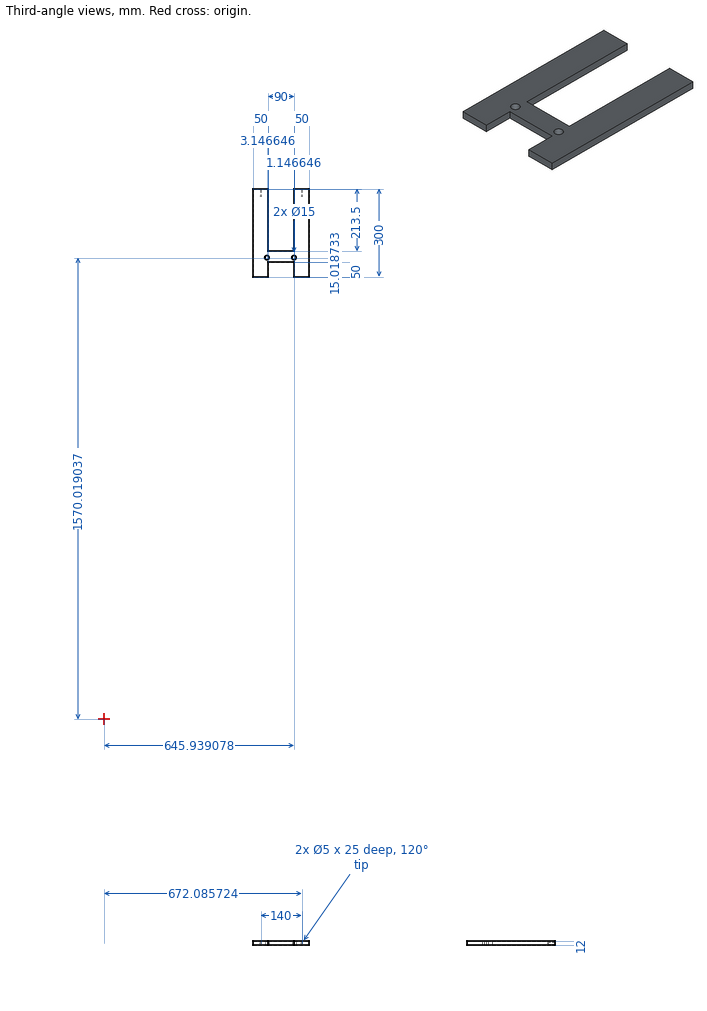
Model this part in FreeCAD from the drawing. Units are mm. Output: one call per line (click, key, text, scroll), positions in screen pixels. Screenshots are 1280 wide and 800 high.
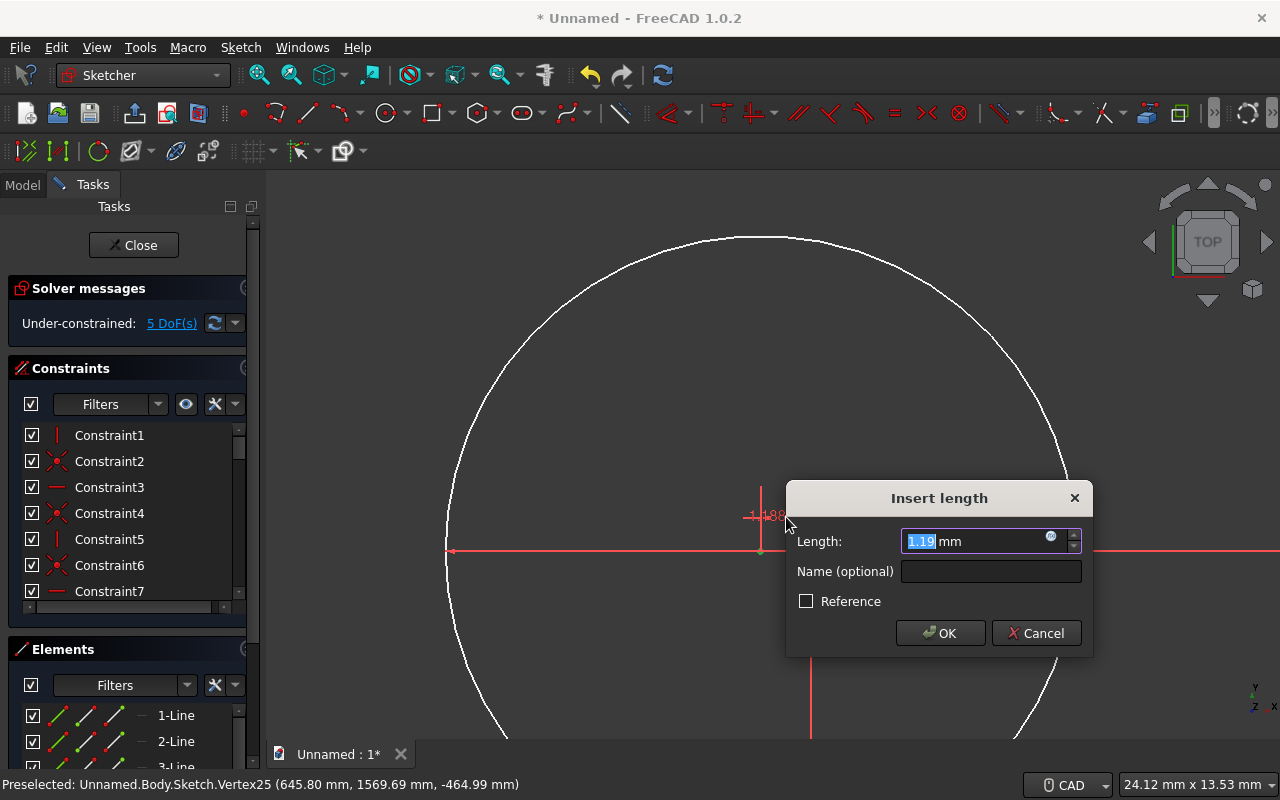
text(1.146646)
key(Return)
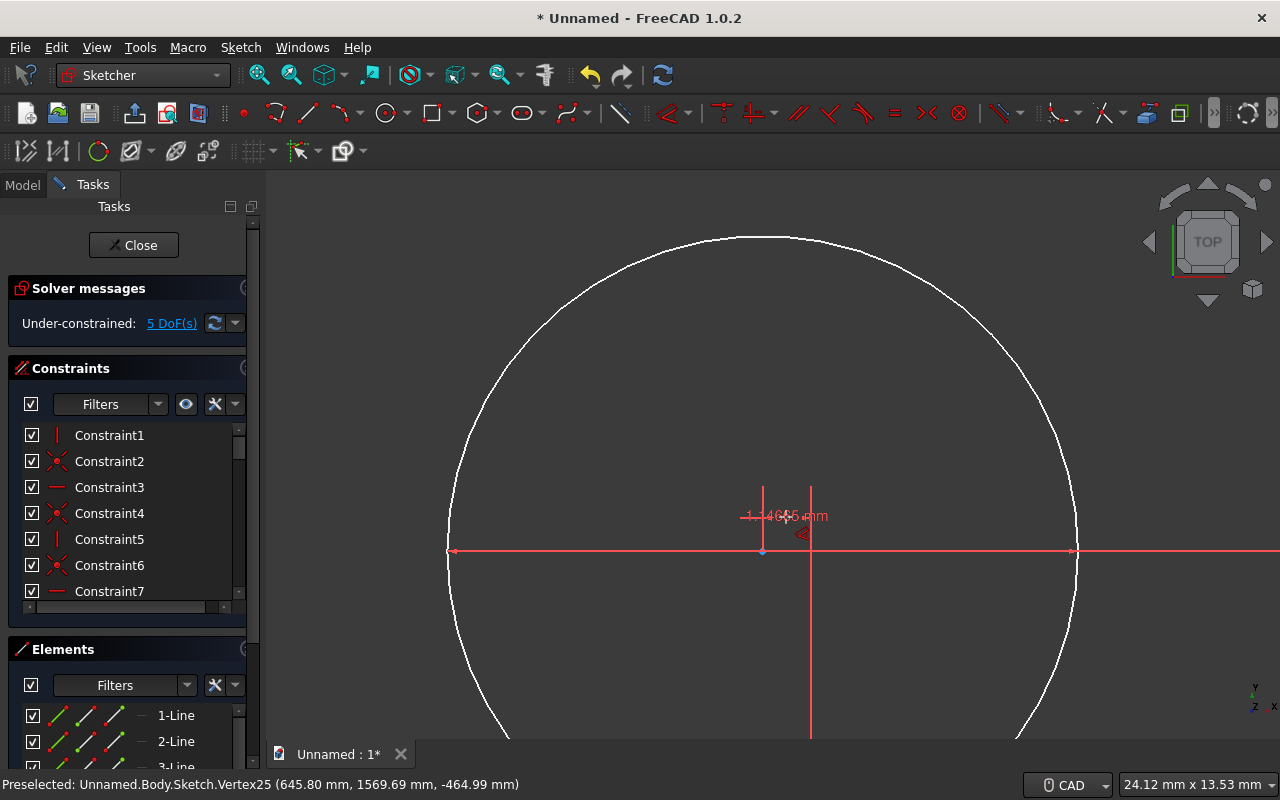
scroll(766, 575, down, 17)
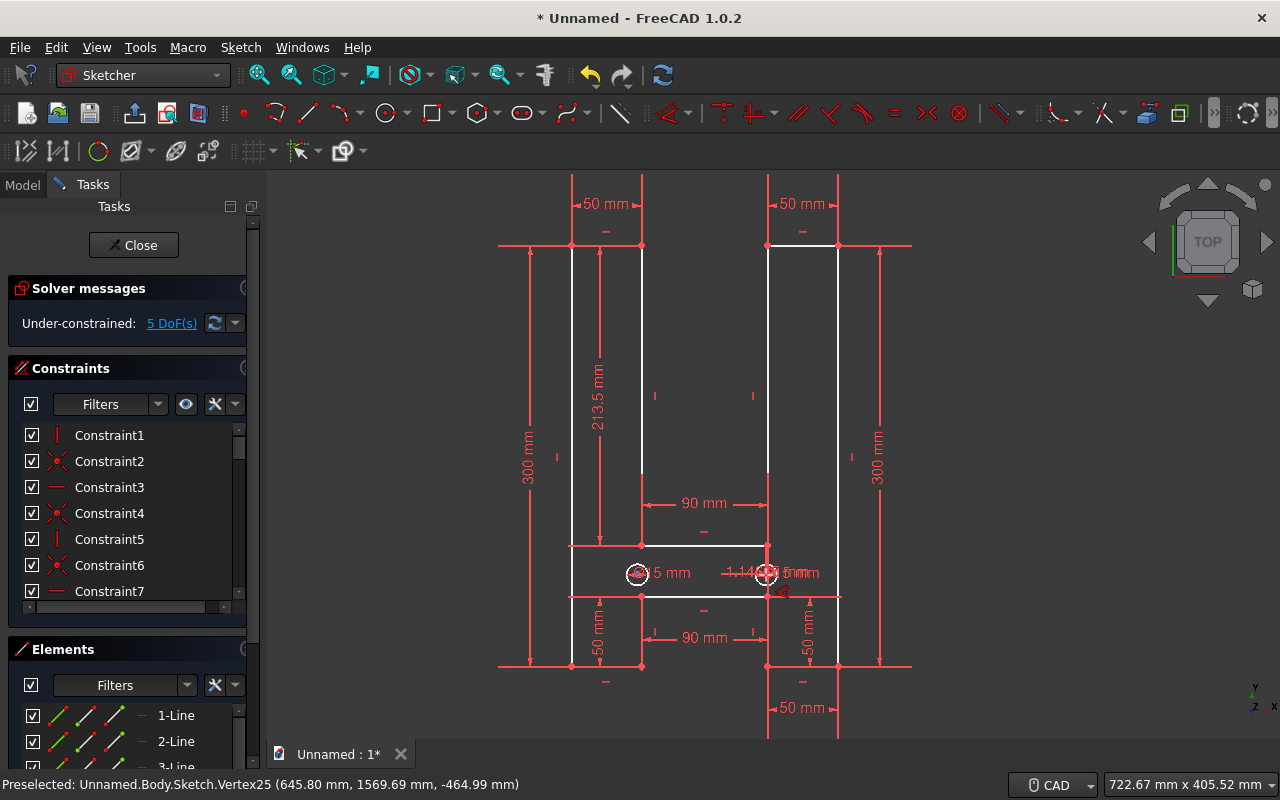
scroll(642, 597, up, 11)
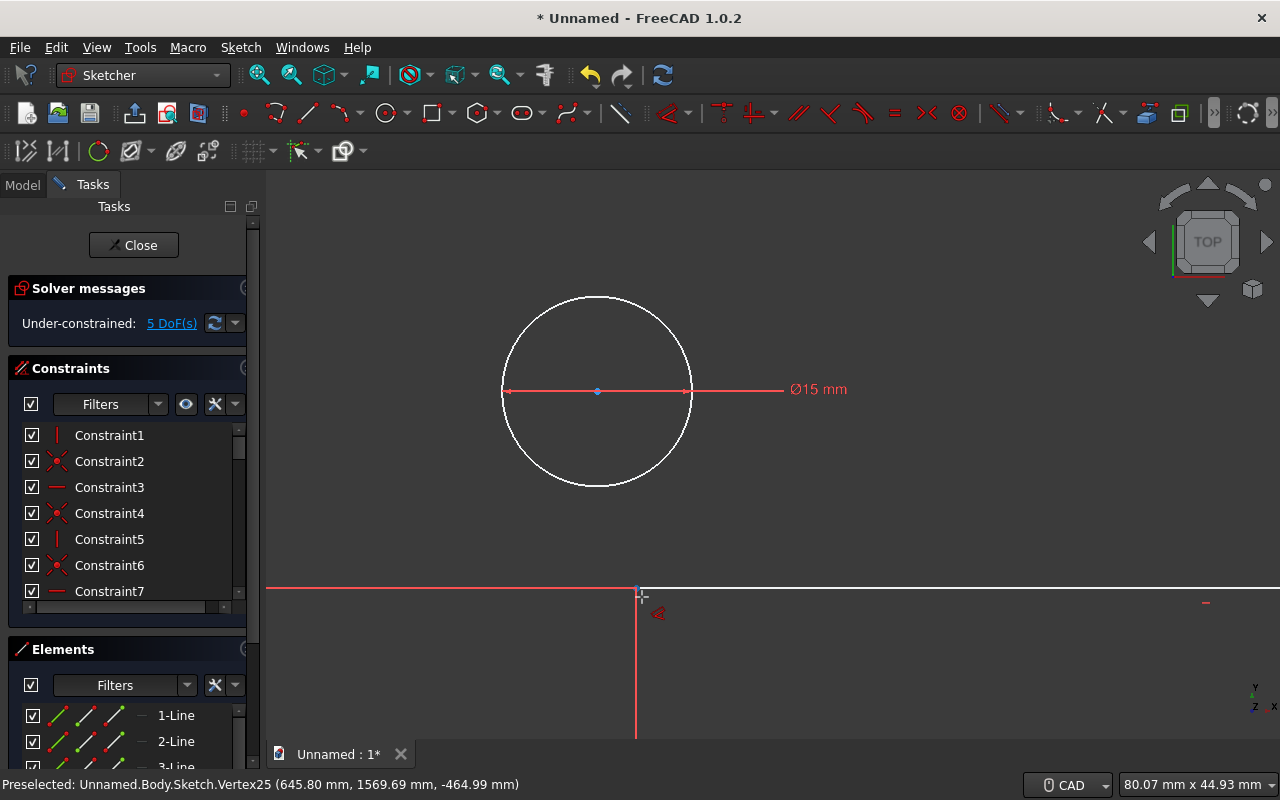
click(636, 588)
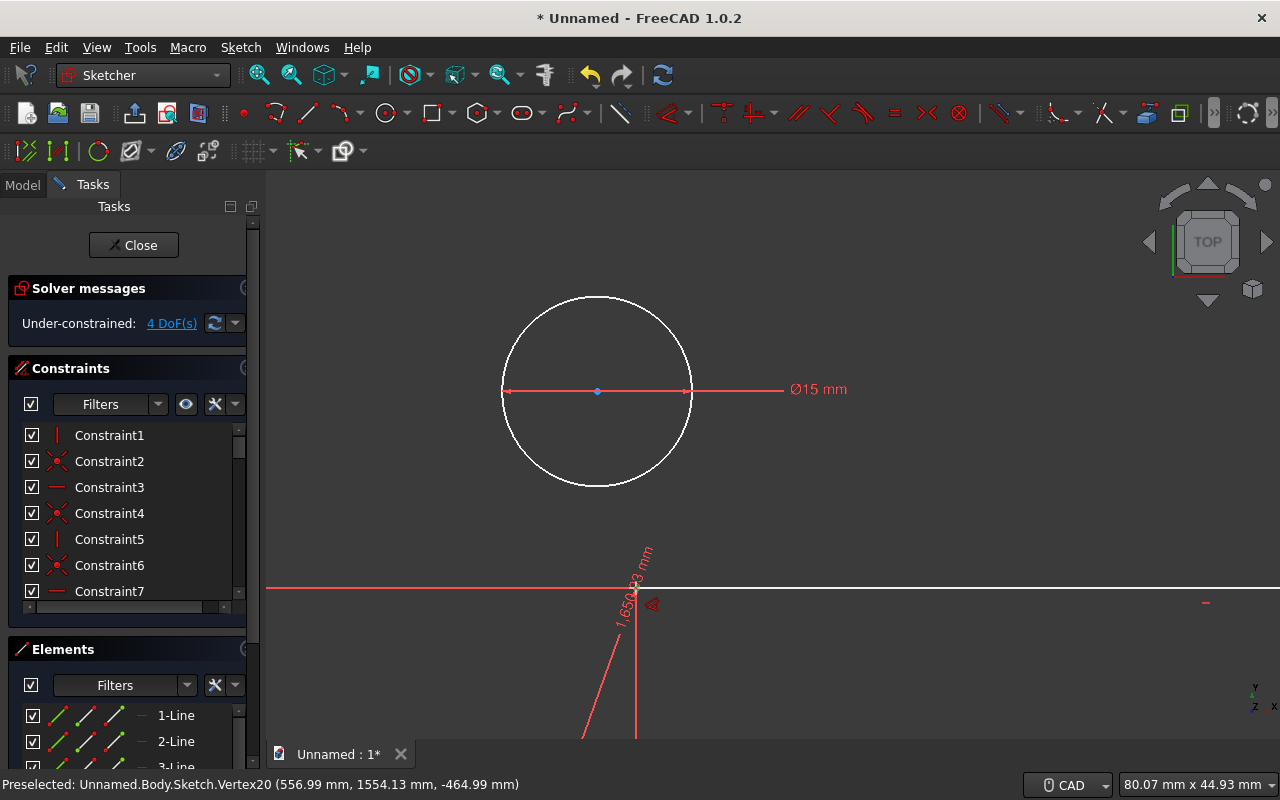
click(597, 391)
click(617, 622)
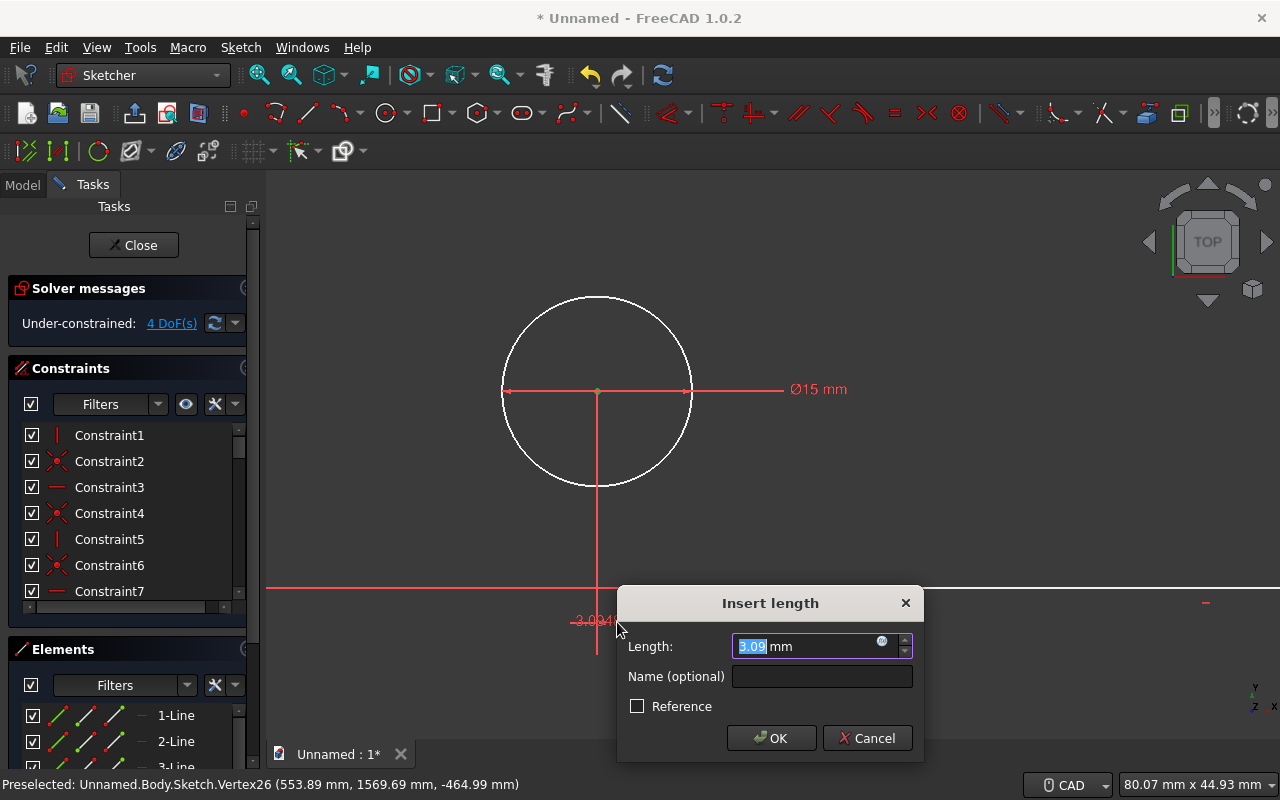
text(3.146646)
key(Return)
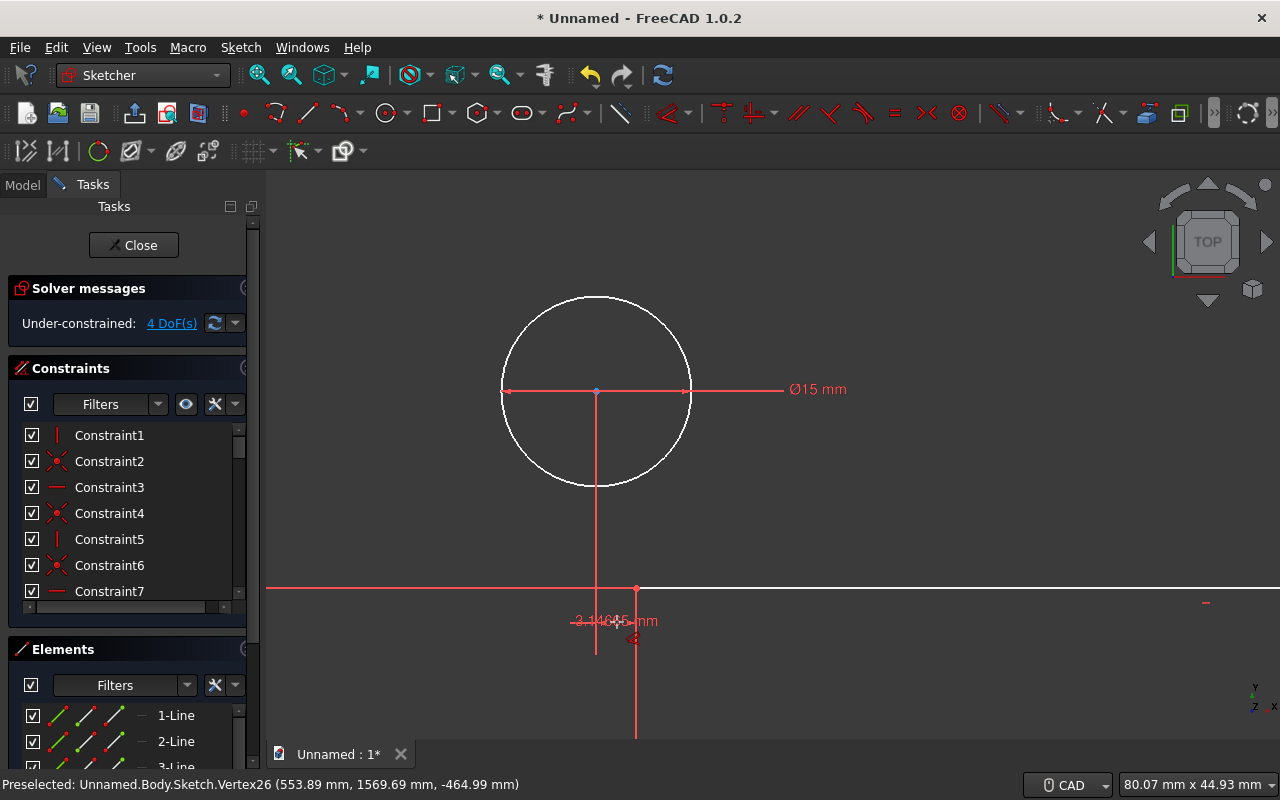
scroll(654, 569, down, 12)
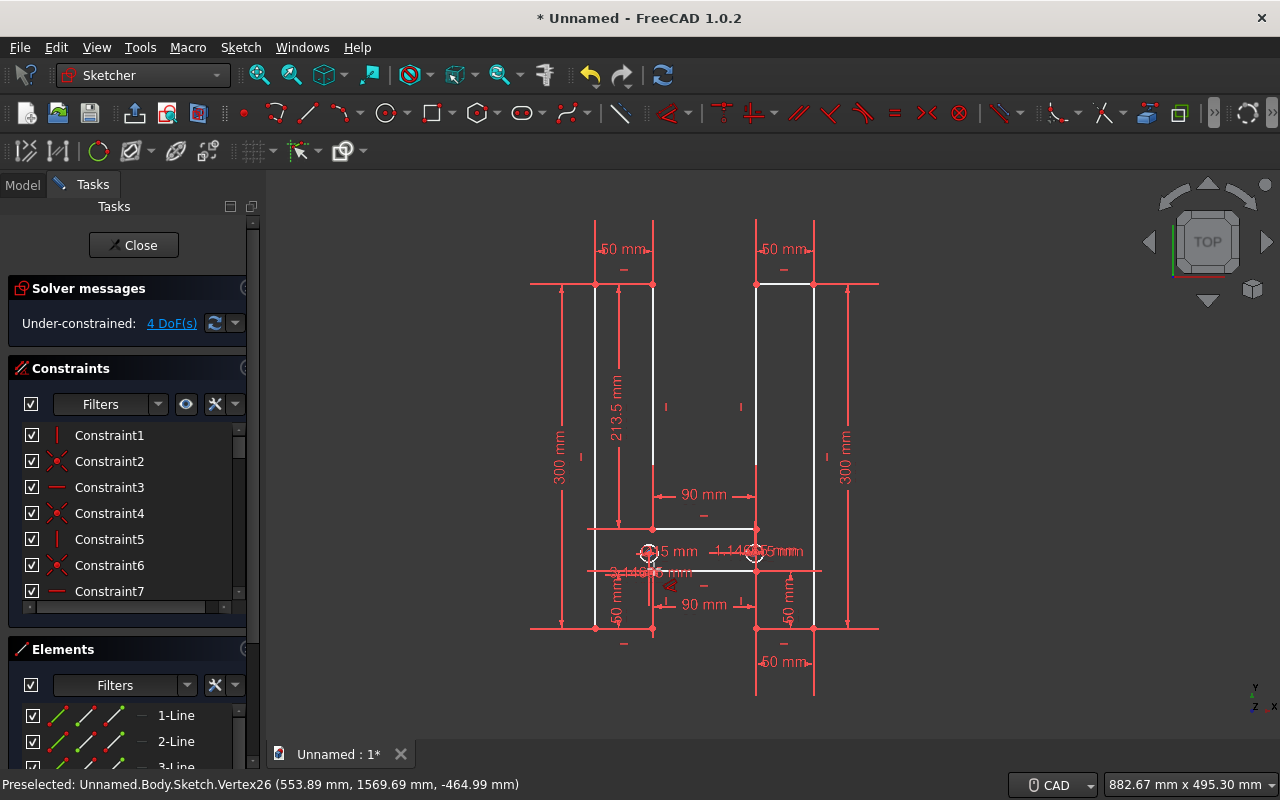
click(755, 554)
click(524, 520)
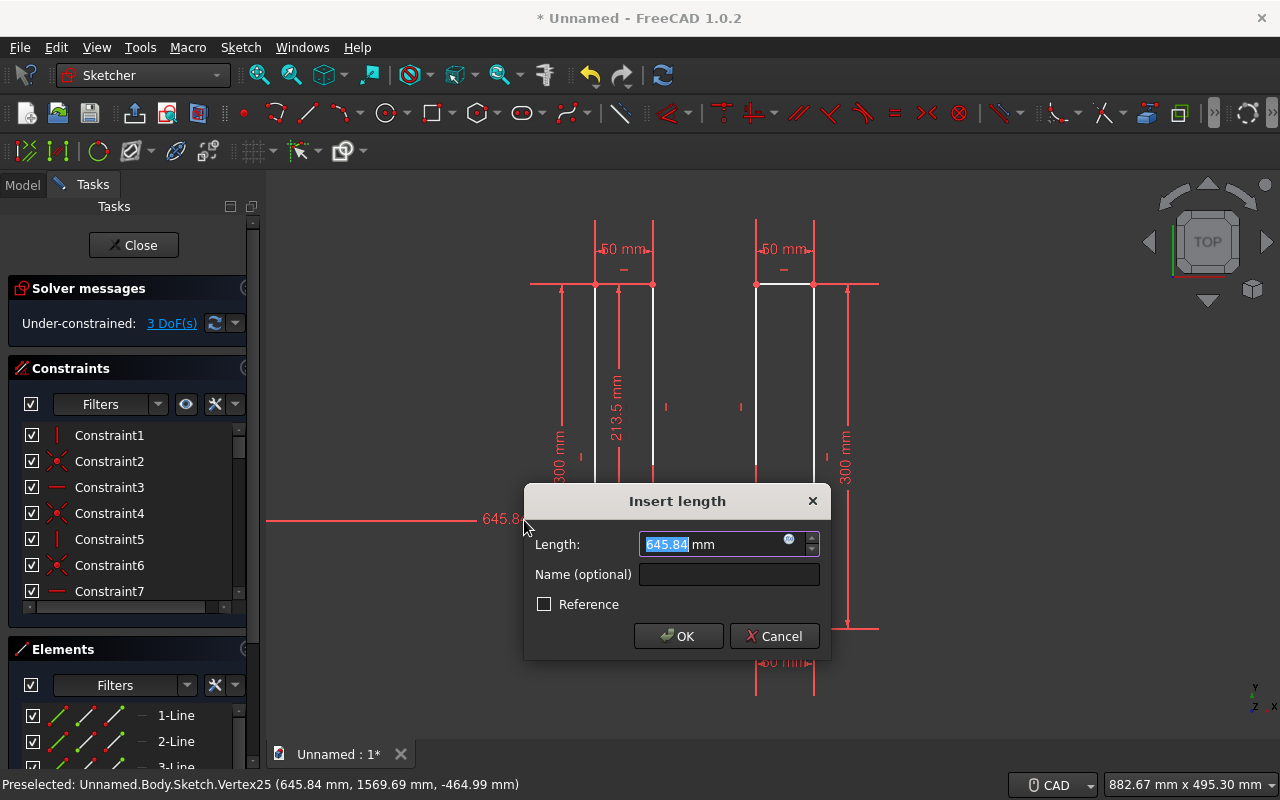
text(645.939078)
key(Return)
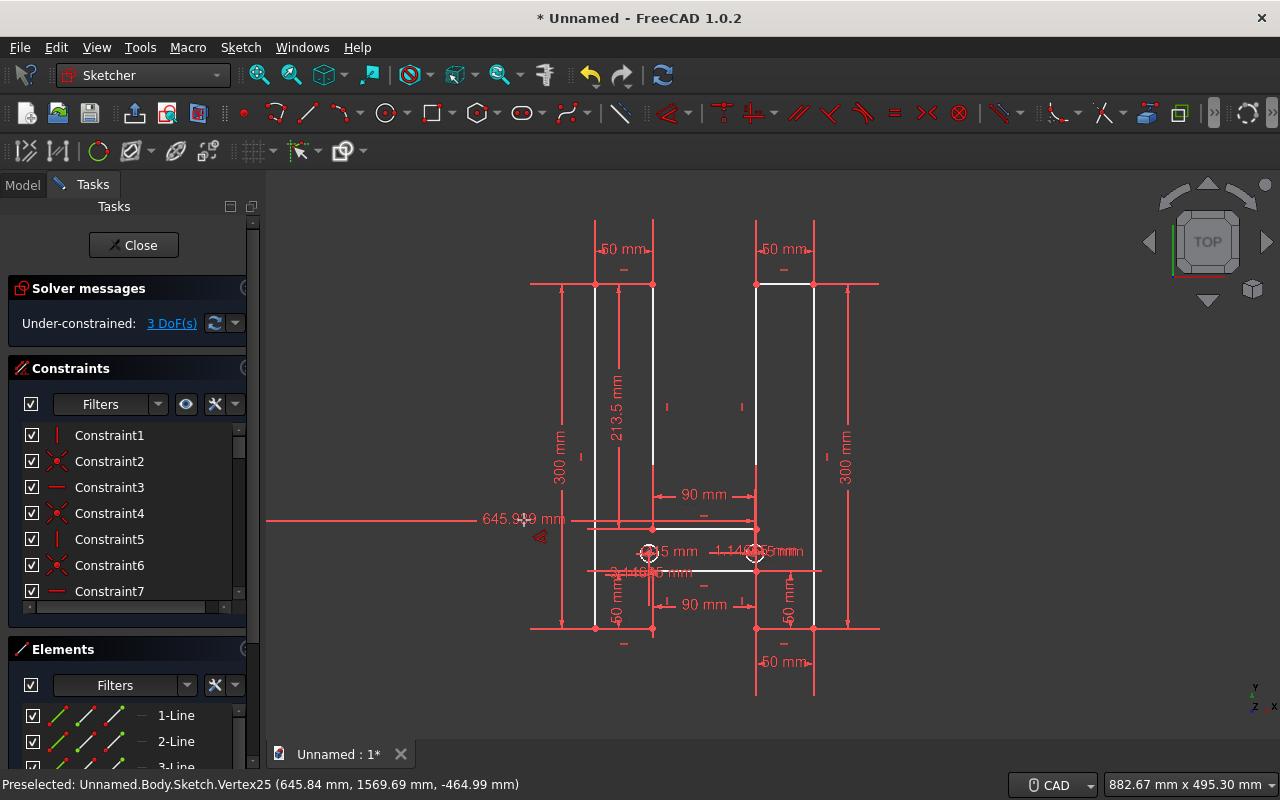
scroll(756, 571, up, 5)